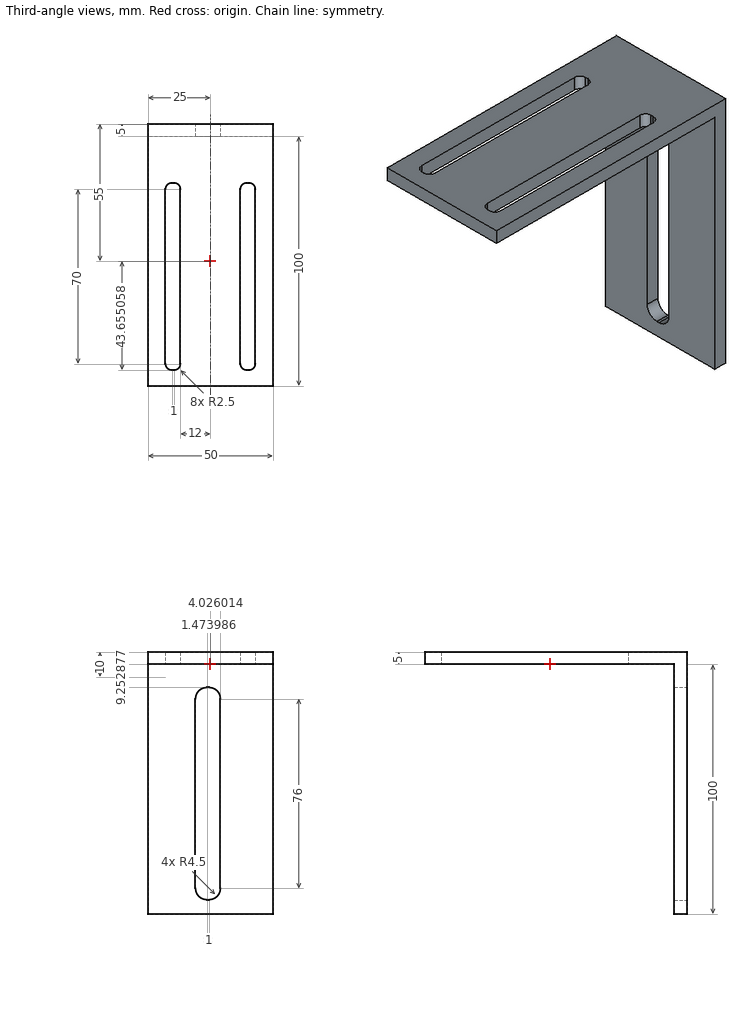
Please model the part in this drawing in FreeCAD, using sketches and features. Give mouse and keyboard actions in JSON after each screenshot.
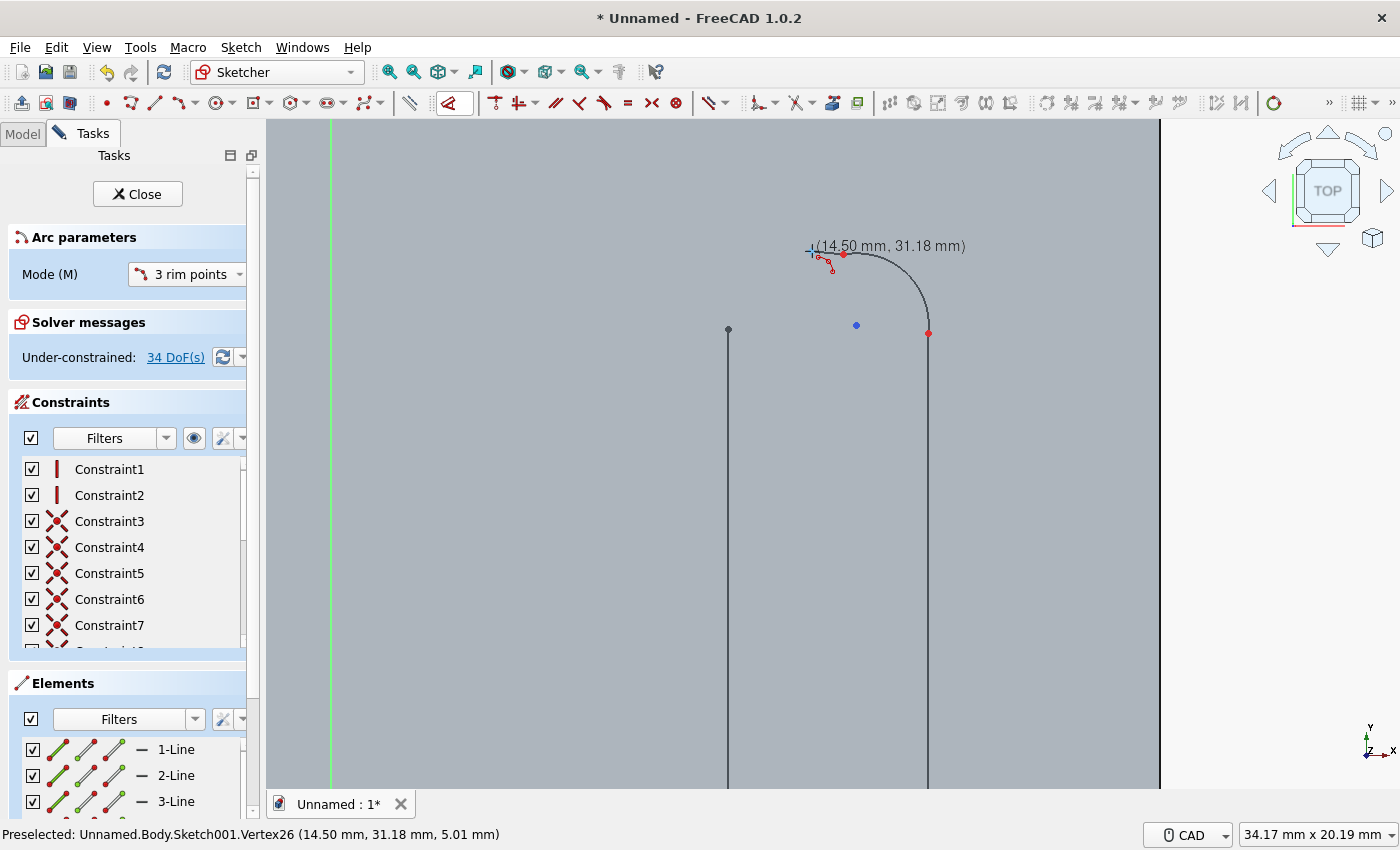
{"action": "scroll", "coordinate": [850, 249], "scroll_direction": "down", "scroll_amount": 9}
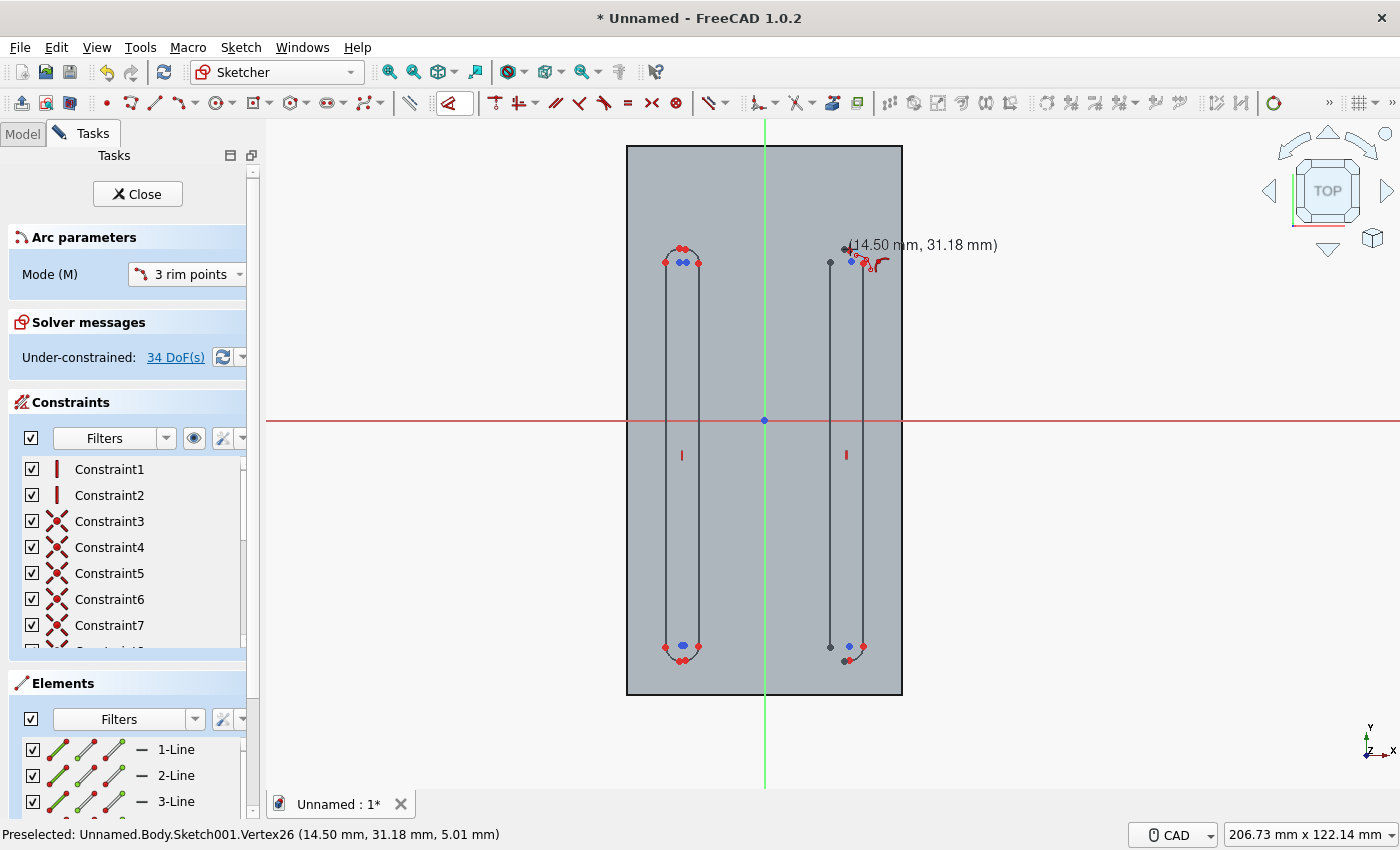
{"action": "left_click", "coordinate": [830, 262]}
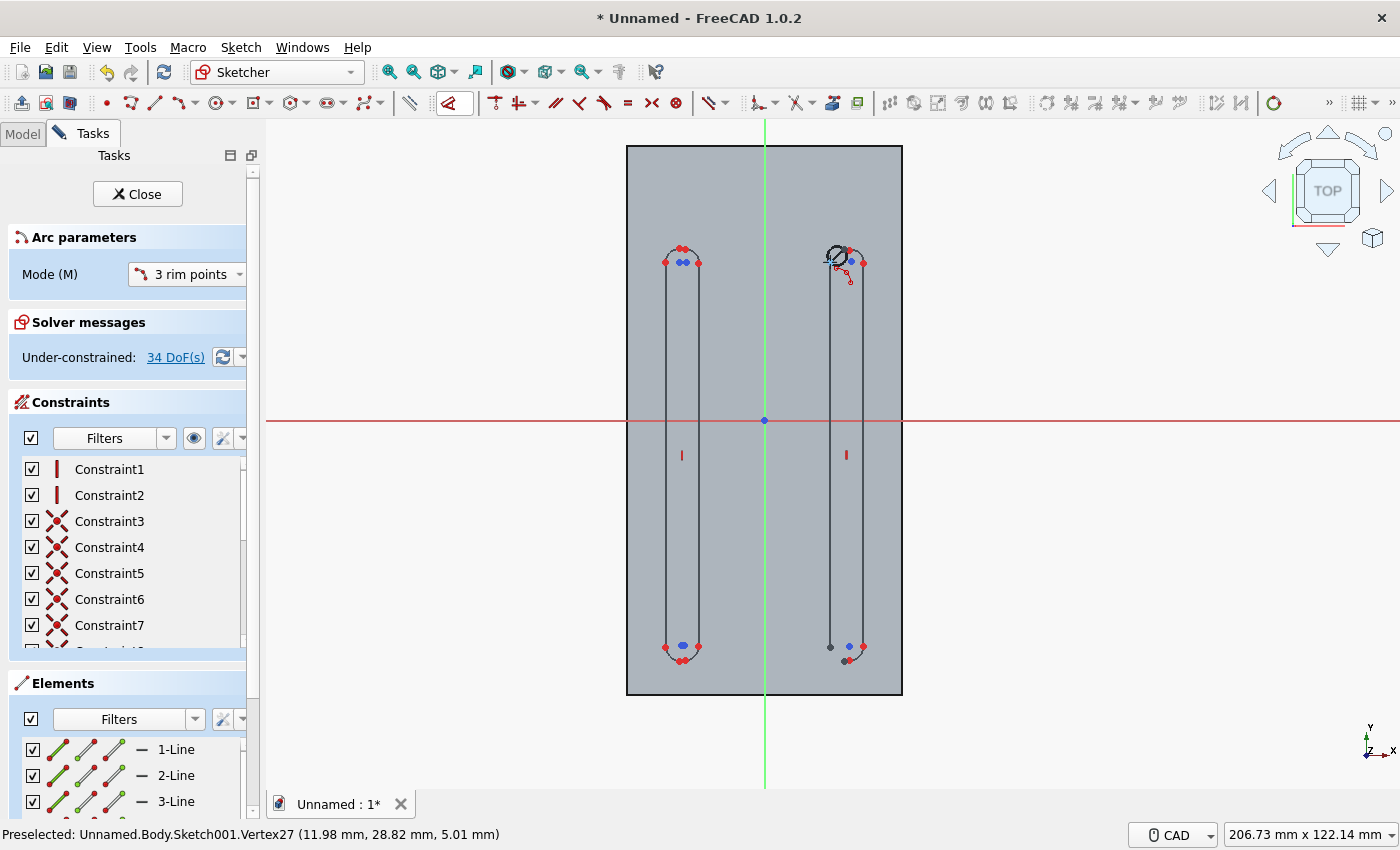
{"action": "scroll", "coordinate": [834, 253], "scroll_direction": "up", "scroll_amount": 7}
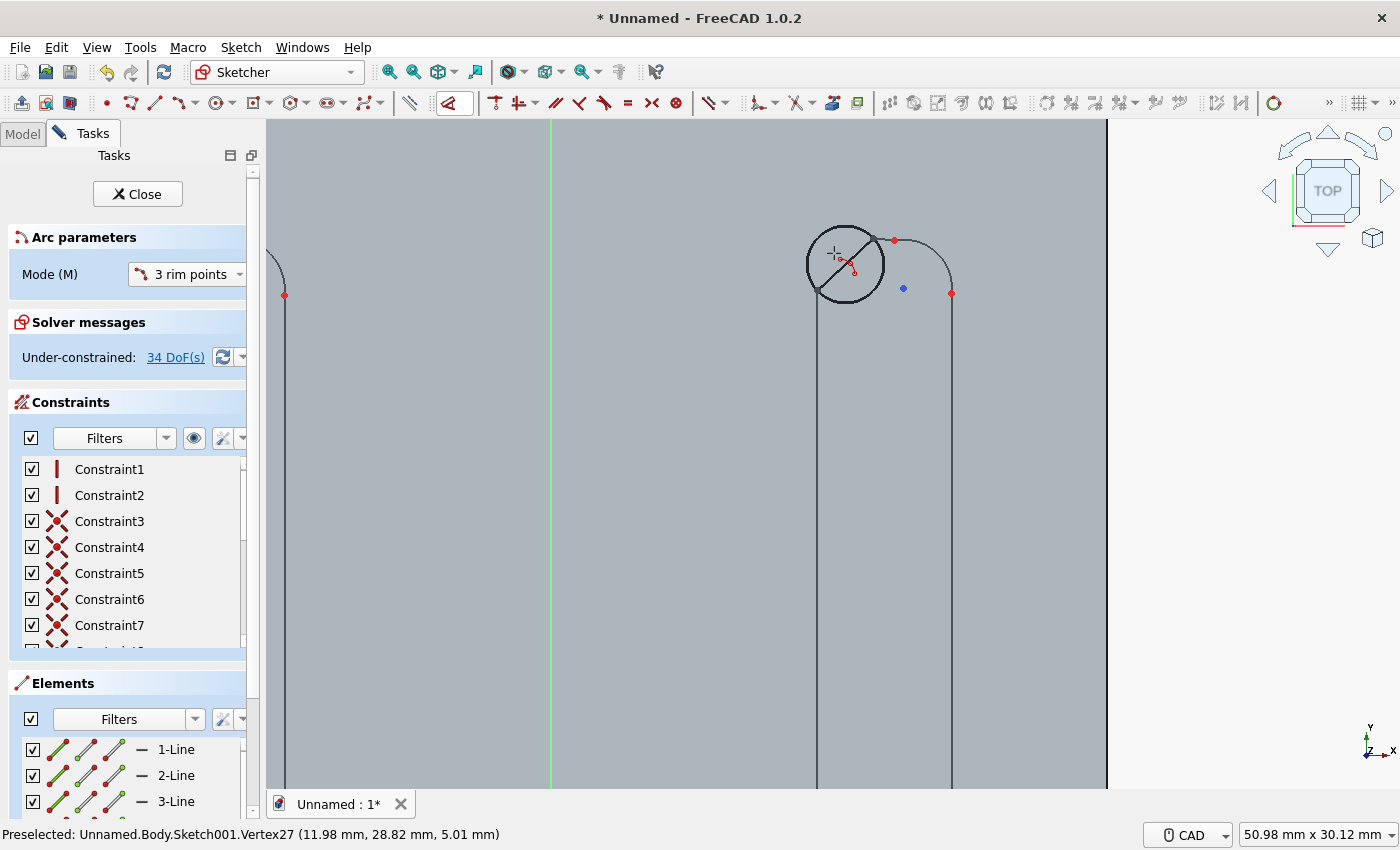
{"action": "left_click", "coordinate": [834, 251]}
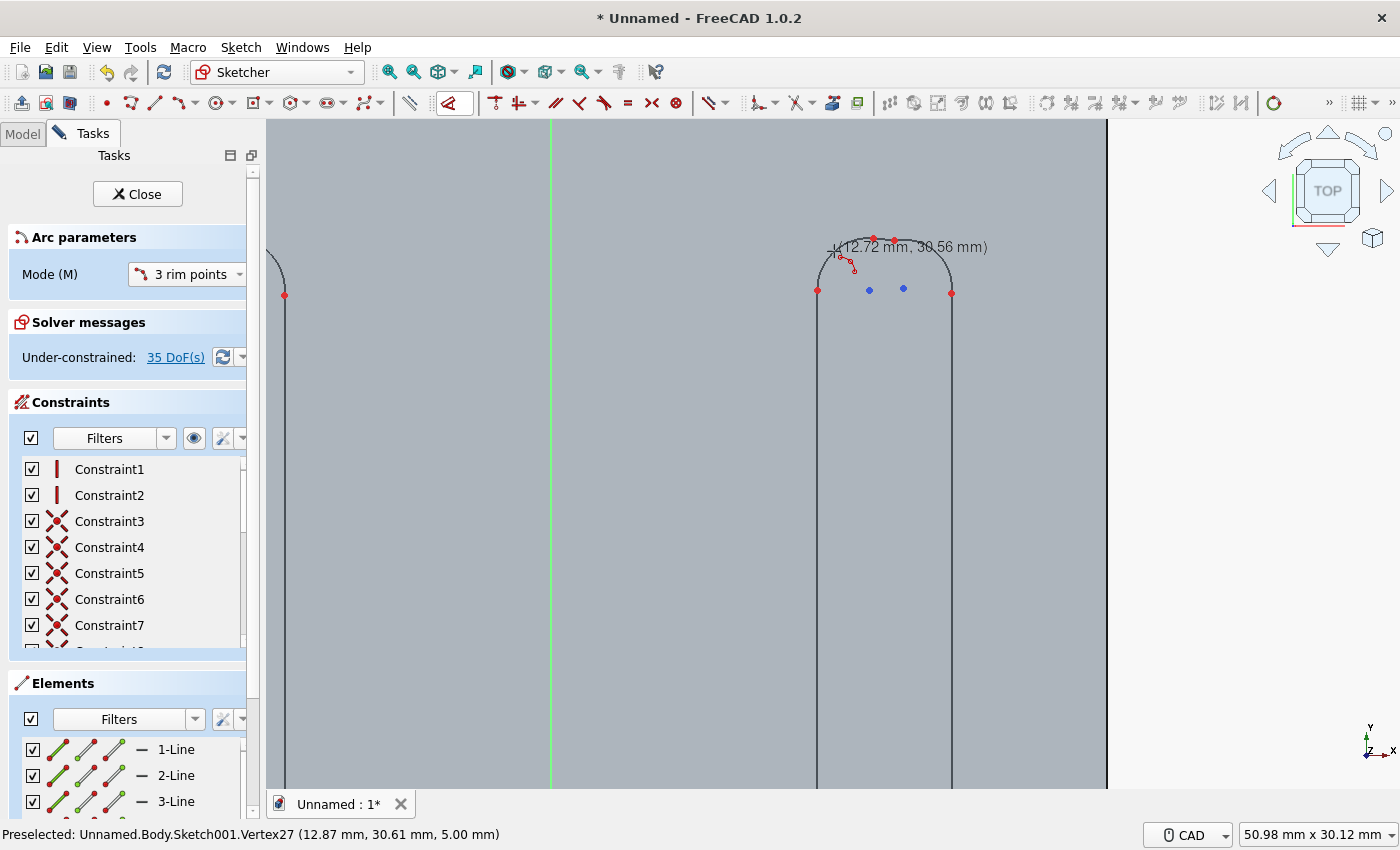
{"action": "scroll", "coordinate": [834, 253], "scroll_direction": "down", "scroll_amount": 7}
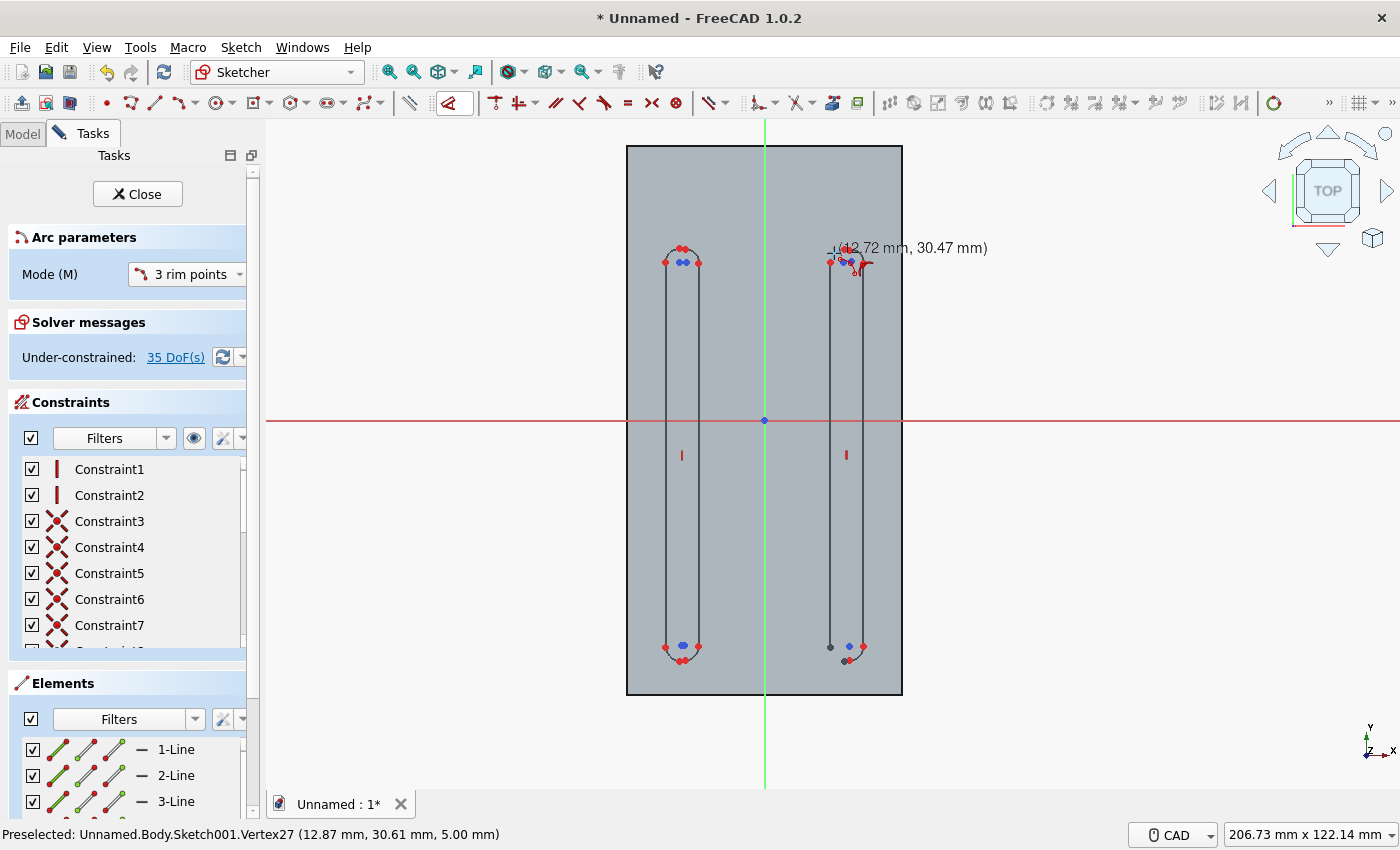
{"action": "left_click", "coordinate": [830, 647]}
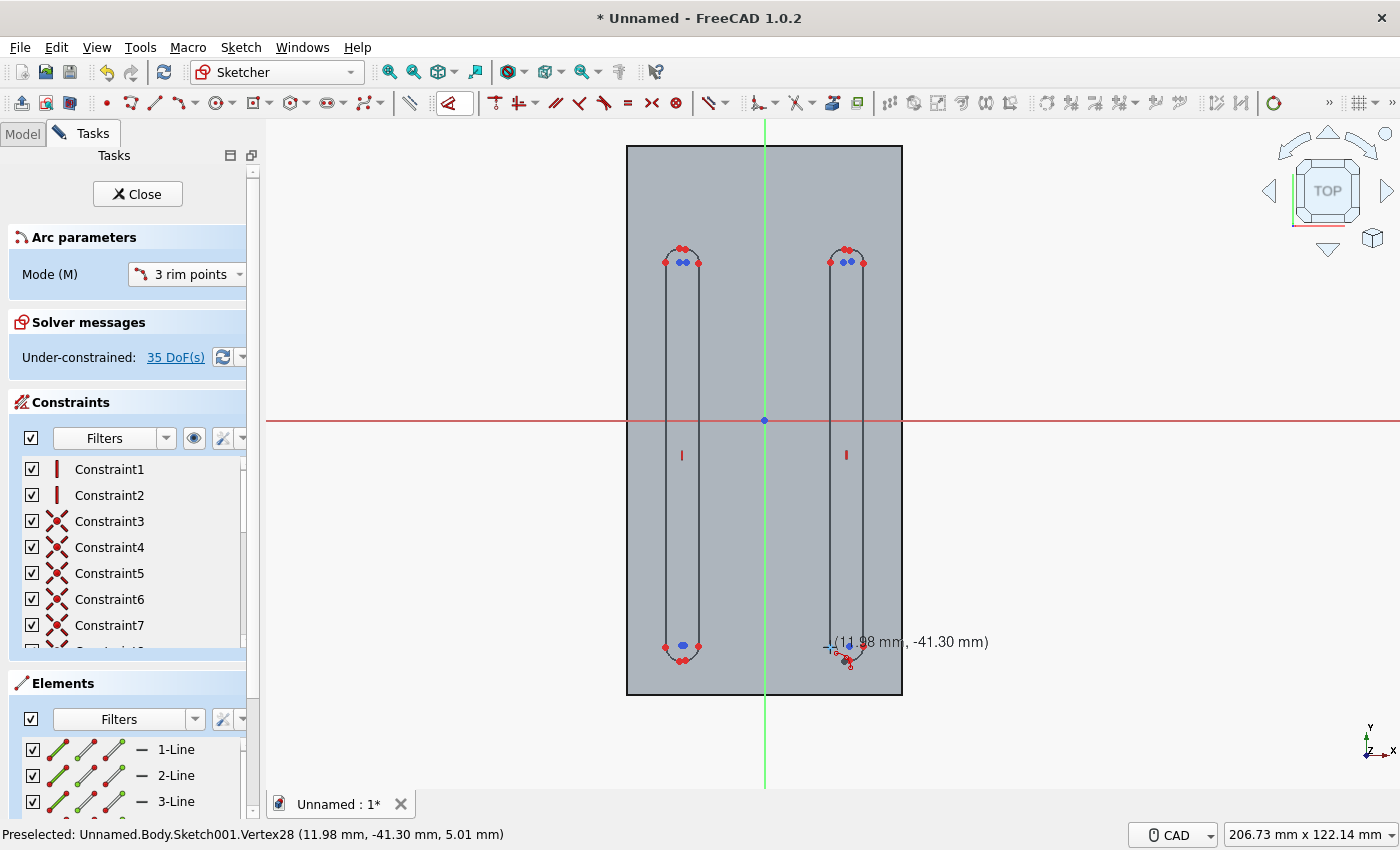
{"action": "scroll", "coordinate": [844, 660], "scroll_direction": "up", "scroll_amount": 9}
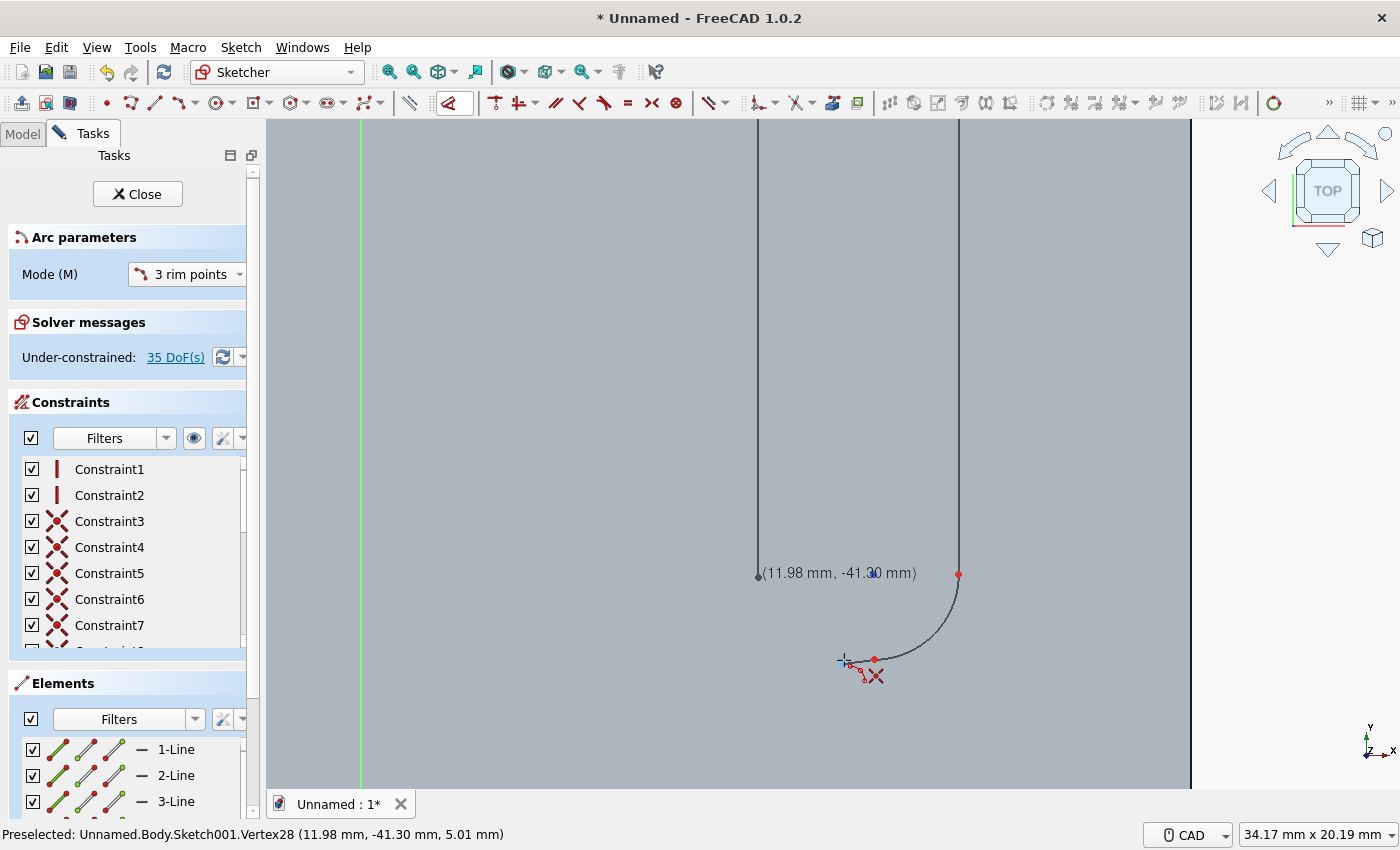
{"action": "left_click", "coordinate": [842, 664]}
{"action": "left_click", "coordinate": [784, 632]}
{"action": "key", "text": "Escape"}